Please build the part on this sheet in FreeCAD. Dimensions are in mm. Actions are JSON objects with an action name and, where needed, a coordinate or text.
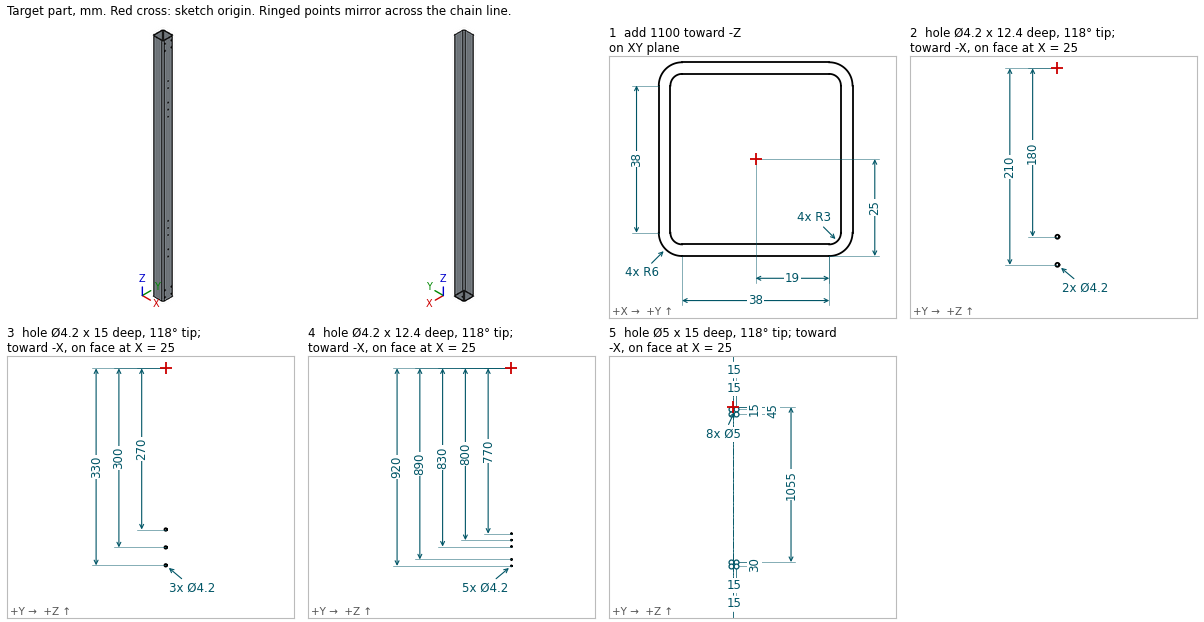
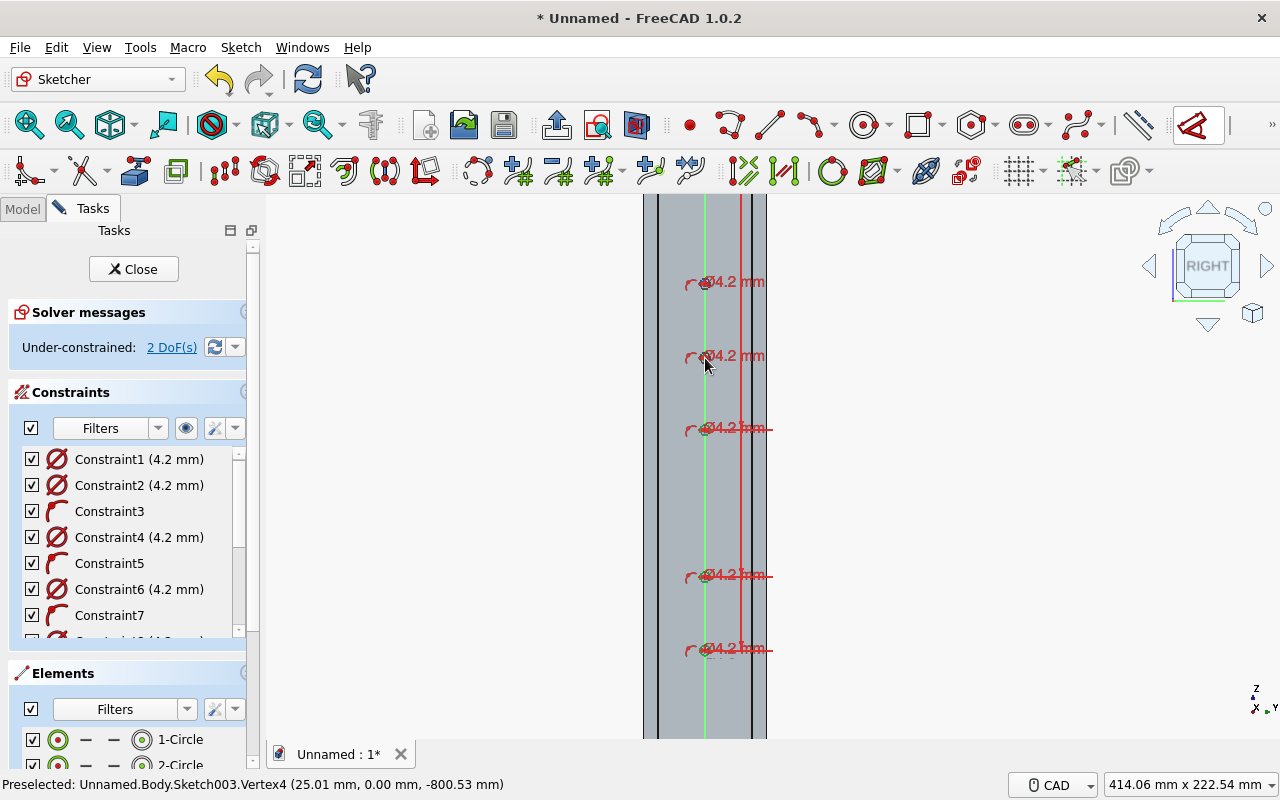
{"action": "left_click", "coordinate": [1218, 126]}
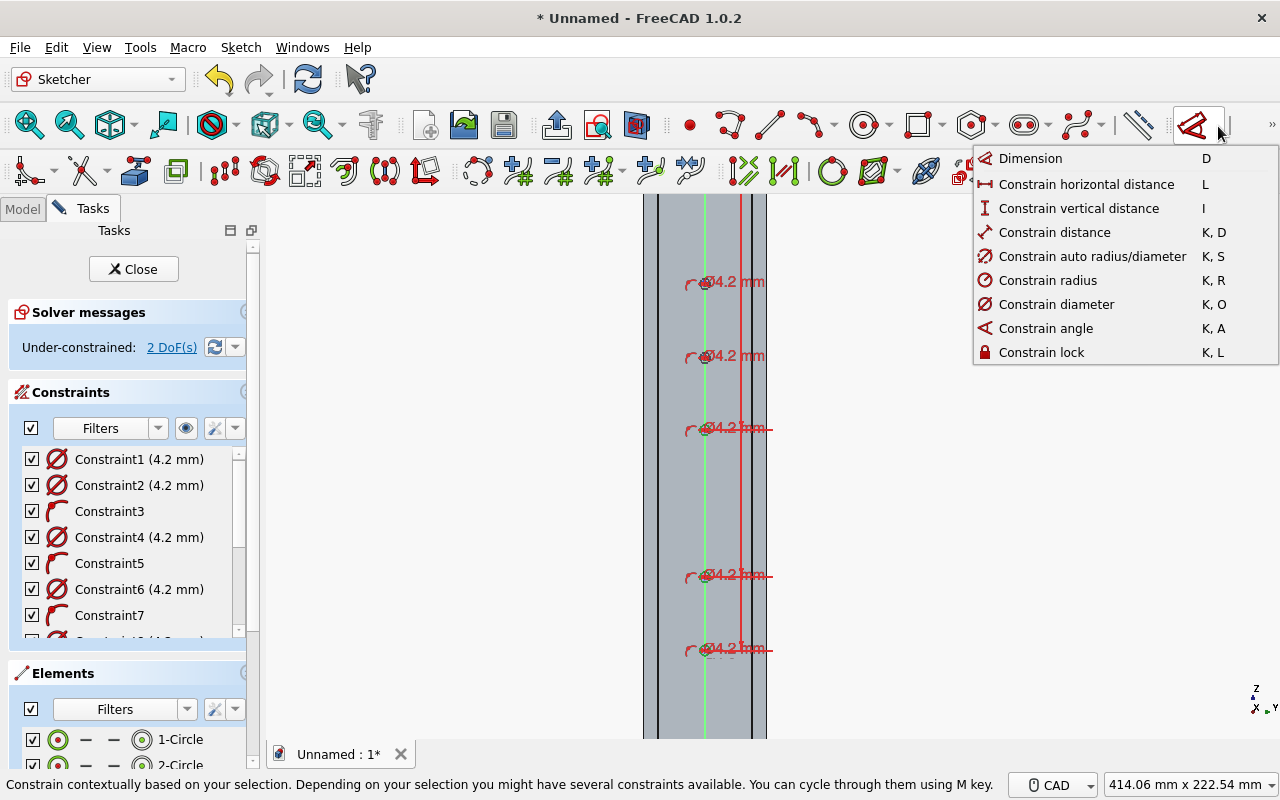
{"action": "left_click", "coordinate": [1126, 208]}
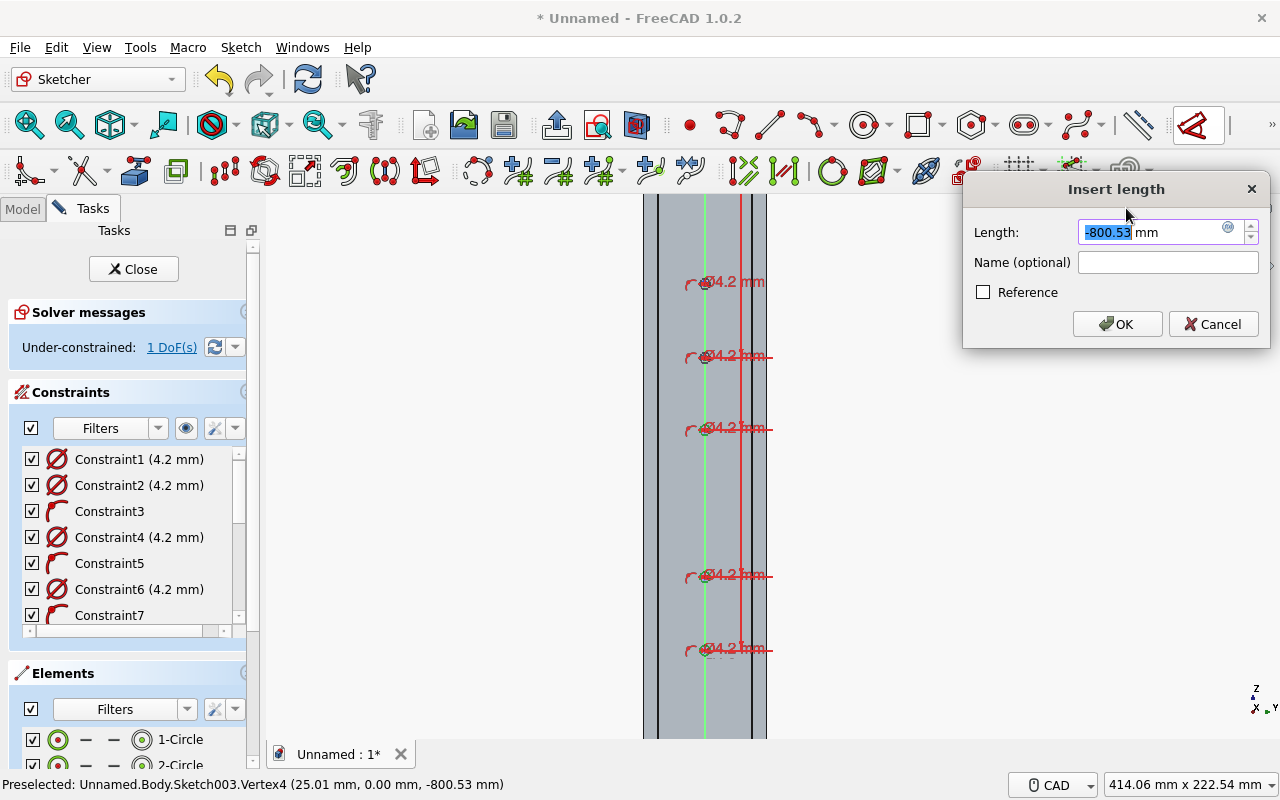
{"action": "type", "text": "-800"}
{"action": "key", "text": "Return"}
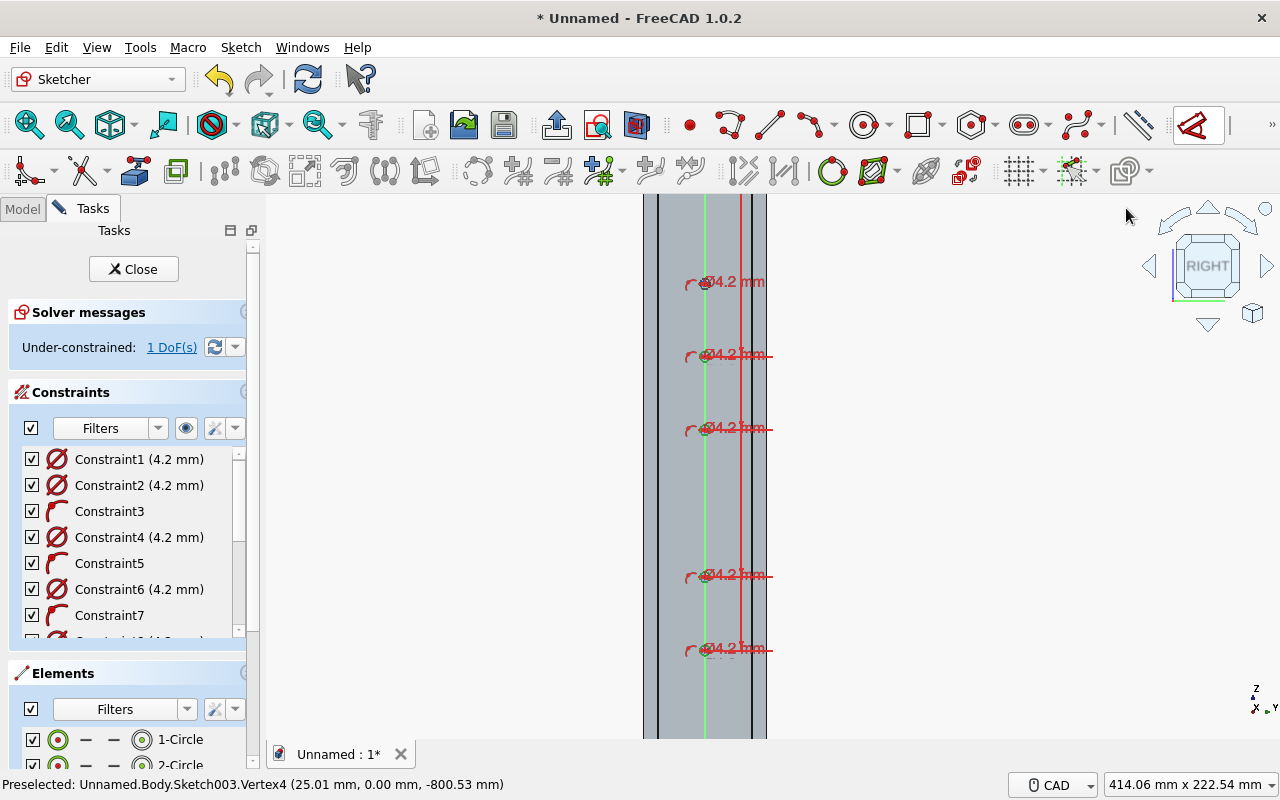
{"action": "left_click", "coordinate": [705, 284]}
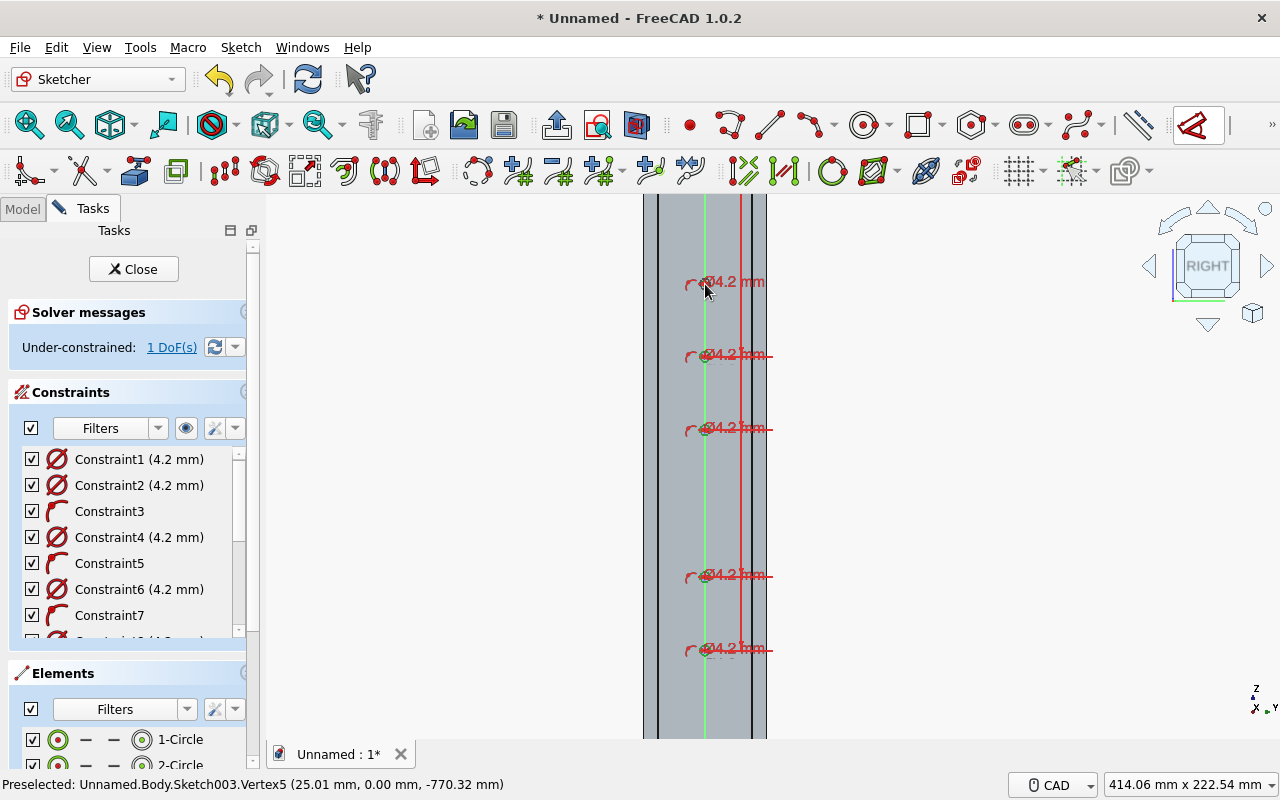
{"action": "left_click", "coordinate": [1218, 126]}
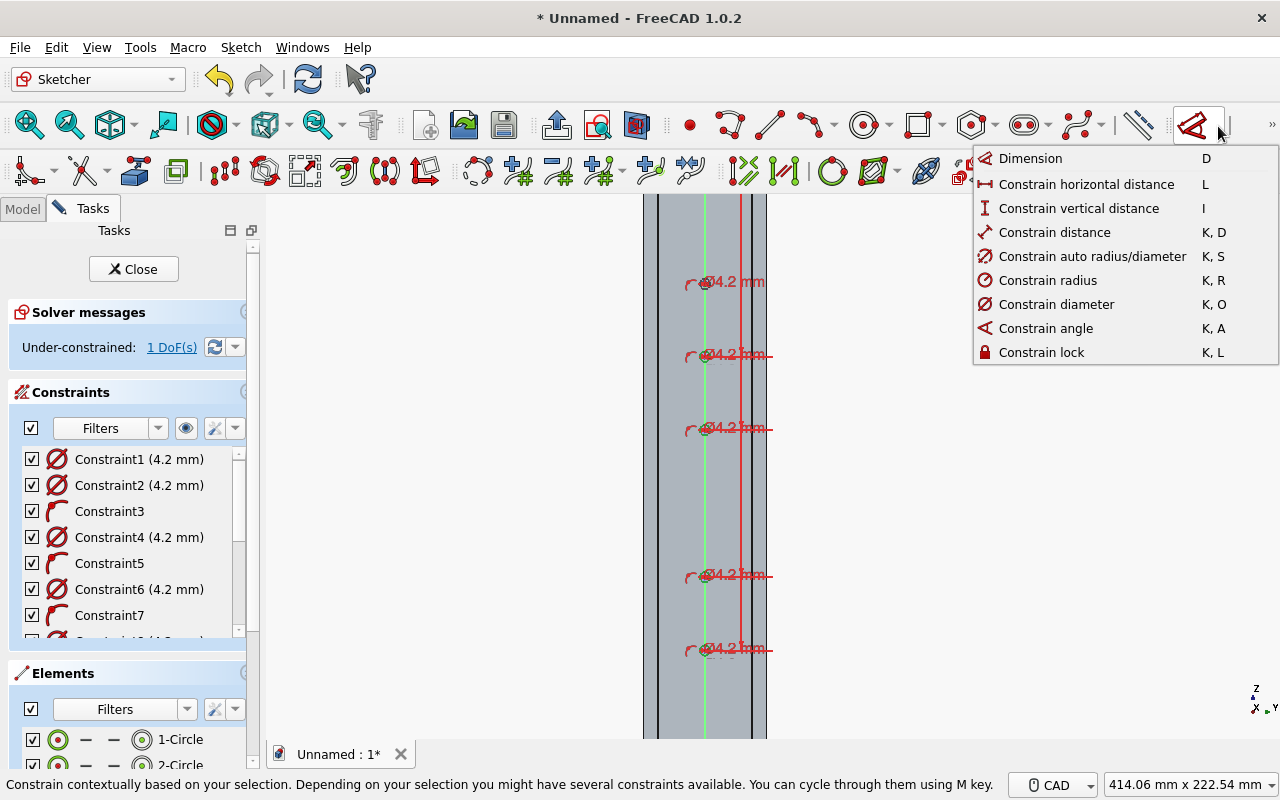
{"action": "left_click", "coordinate": [1126, 208]}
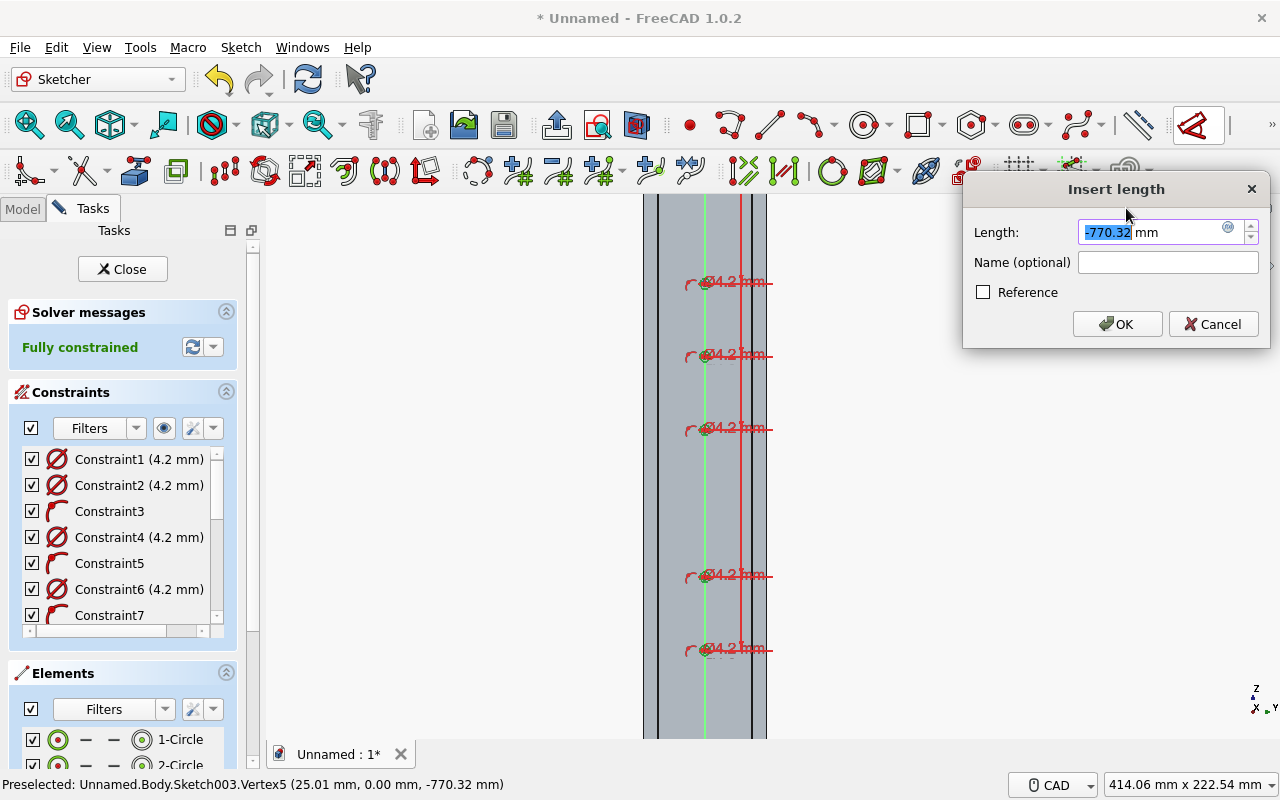
{"action": "type", "text": "-770"}
{"action": "key", "text": "Return"}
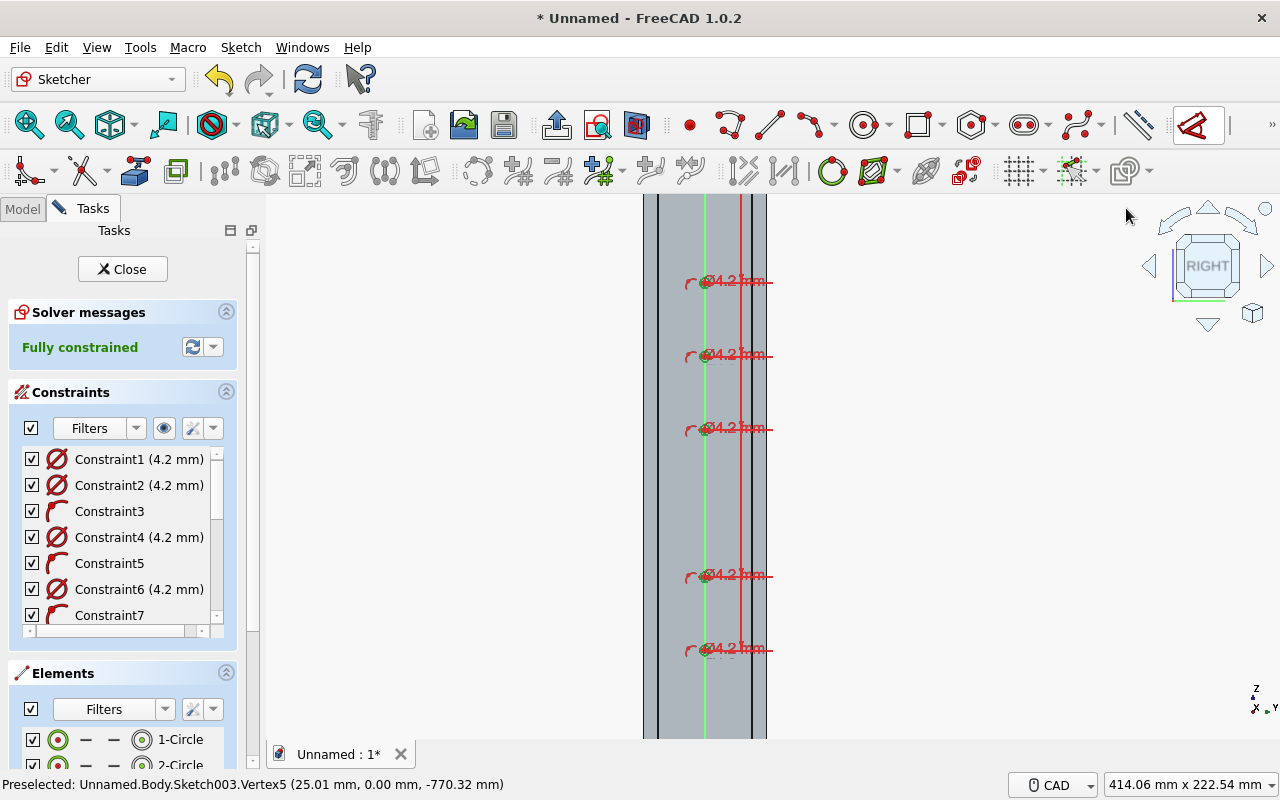
{"action": "left_click", "coordinate": [123, 269]}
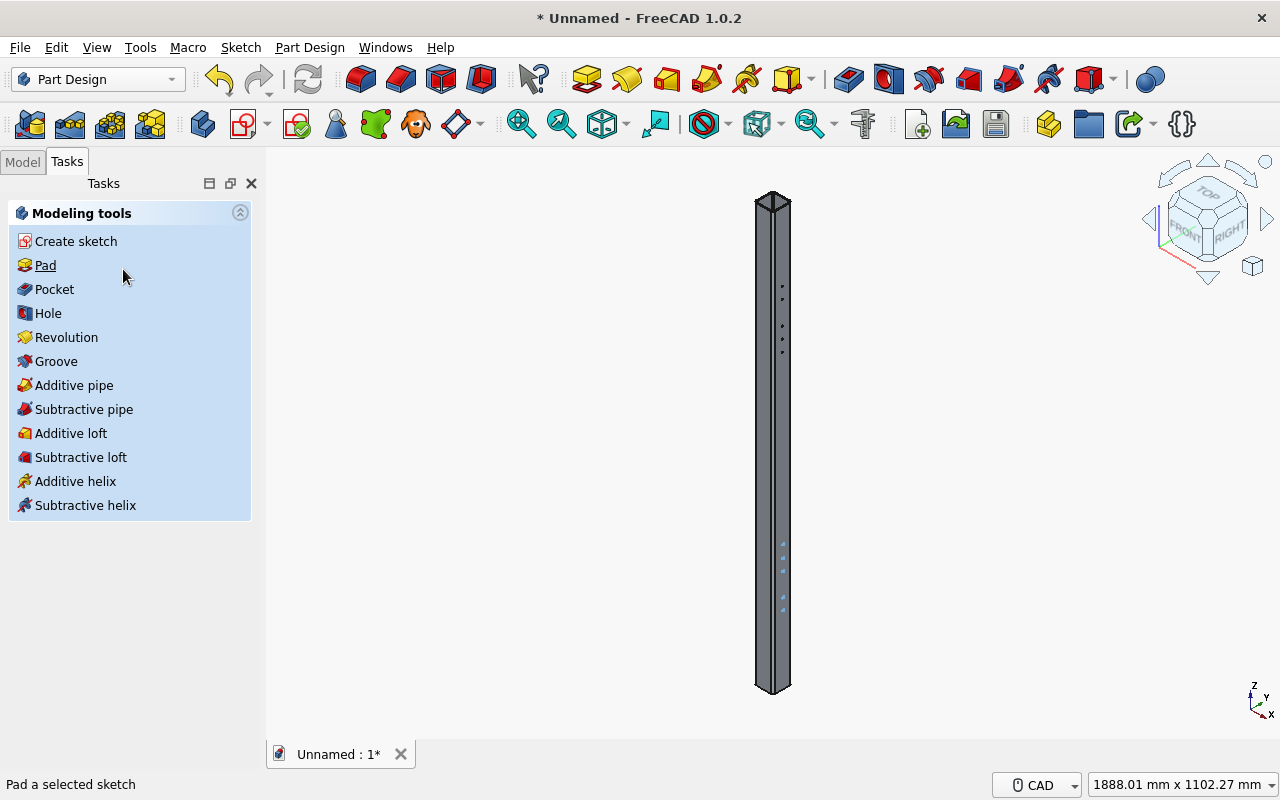
{"action": "left_click", "coordinate": [890, 80]}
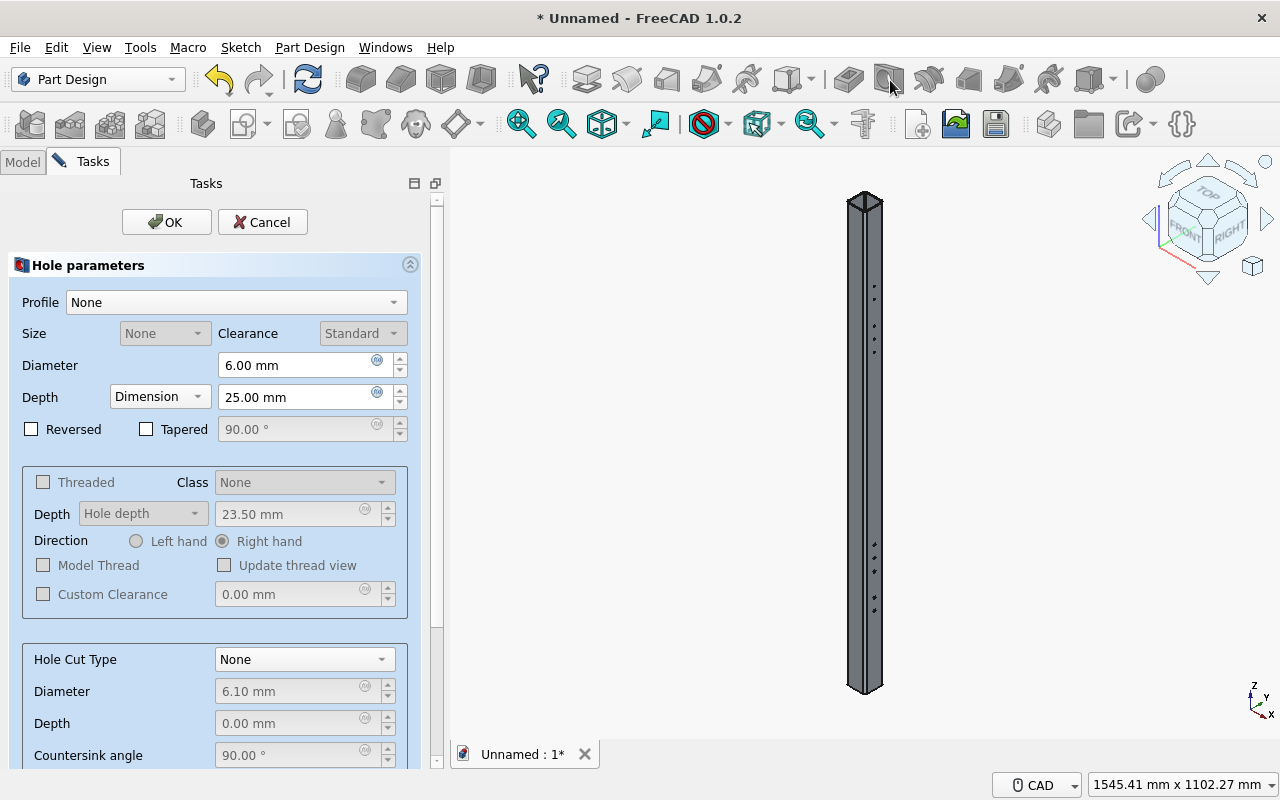
{"action": "triple_click", "coordinate": [305, 365]}